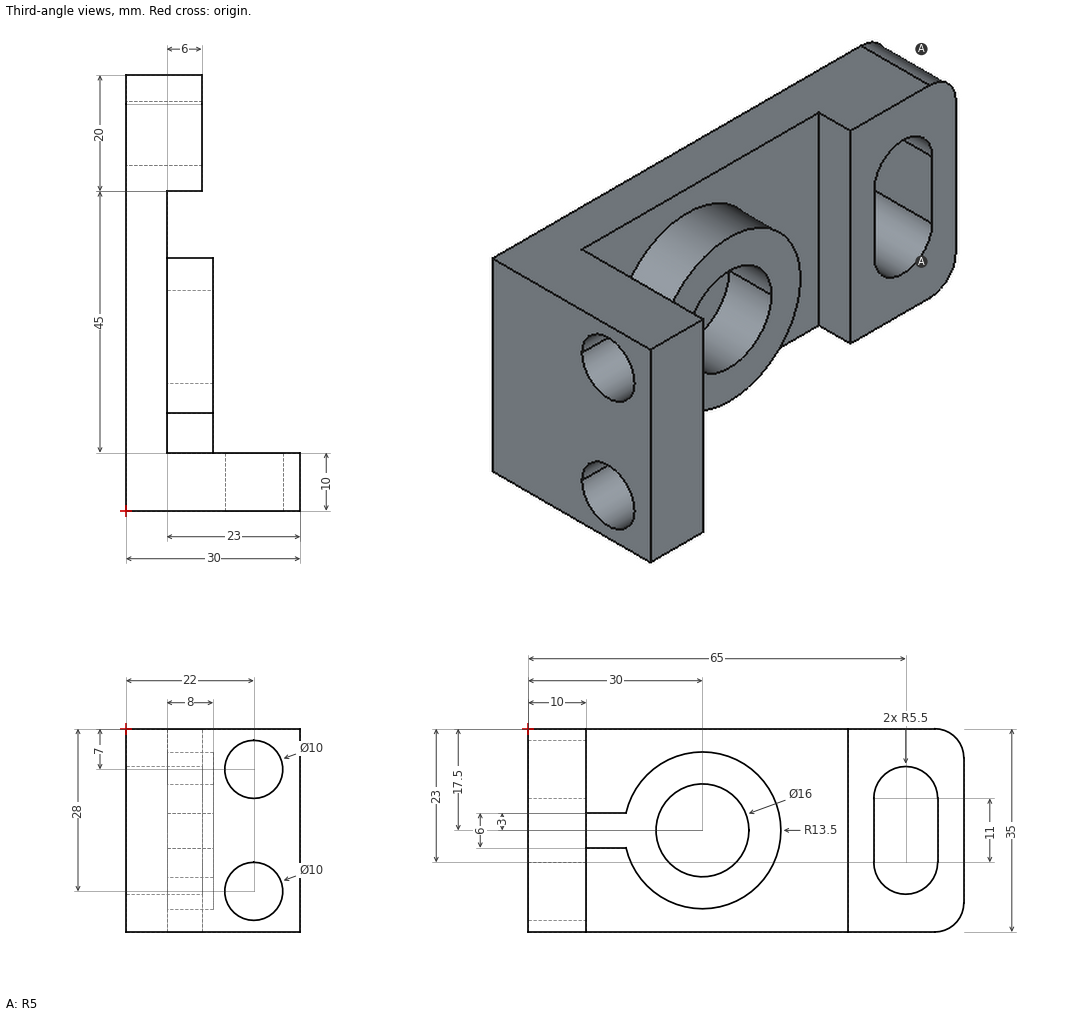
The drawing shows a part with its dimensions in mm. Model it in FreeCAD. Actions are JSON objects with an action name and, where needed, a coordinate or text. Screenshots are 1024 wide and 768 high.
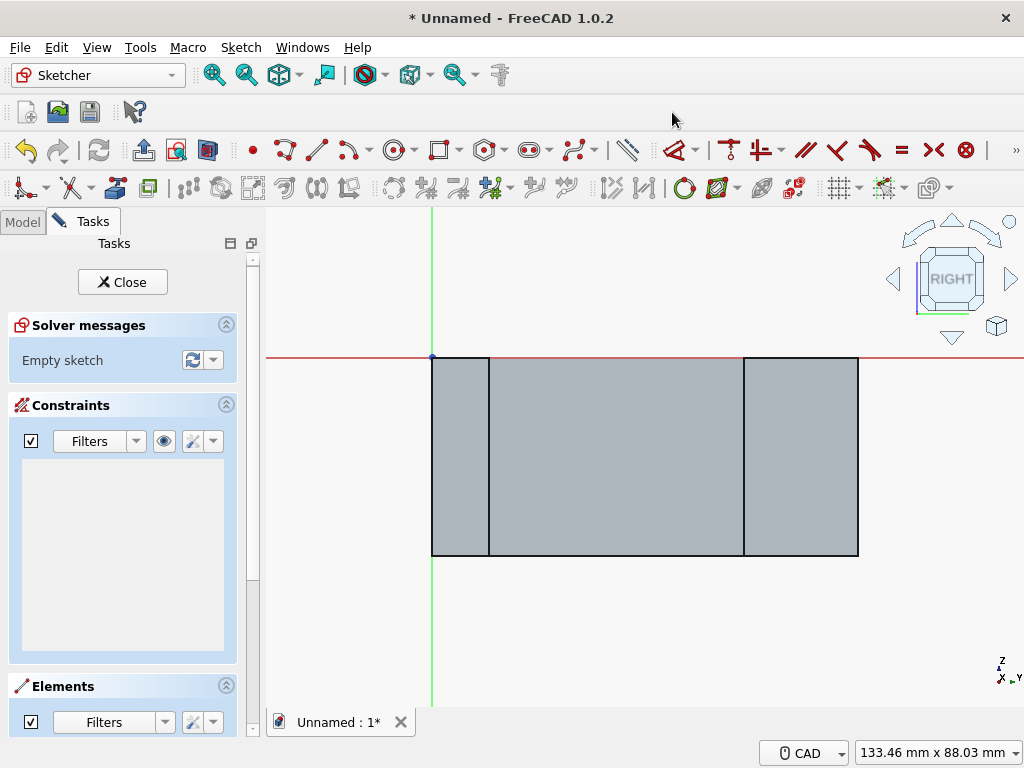
{"action": "scroll", "coordinate": [513, 375], "scroll_direction": "up", "scroll_amount": 2}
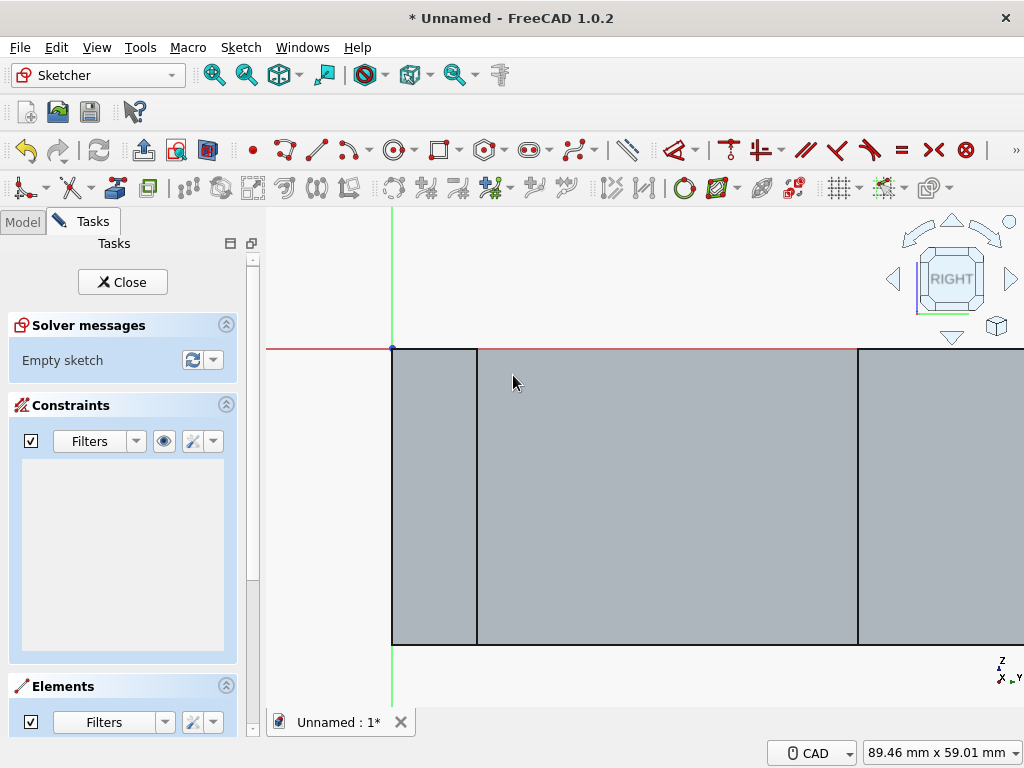
{"action": "left_click", "coordinate": [286, 150]}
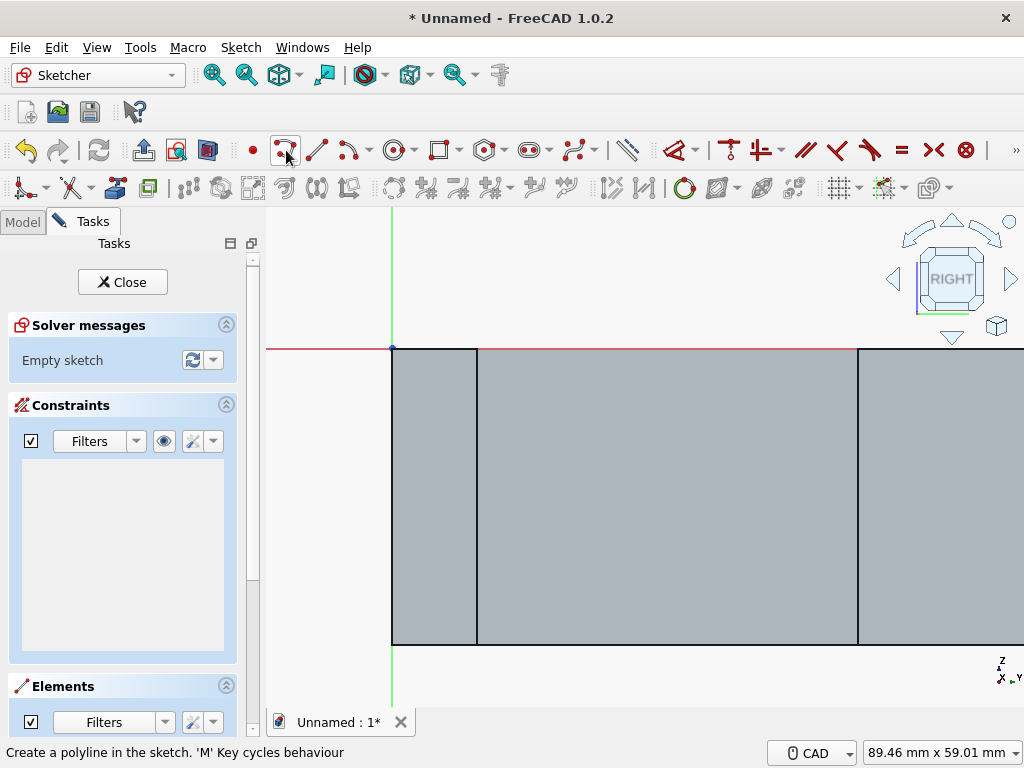
{"action": "left_click", "coordinate": [535, 472]}
{"action": "left_click", "coordinate": [477, 472]}
{"action": "left_click", "coordinate": [477, 523]}
{"action": "left_click", "coordinate": [535, 523]}
{"action": "right_click", "coordinate": [535, 523]}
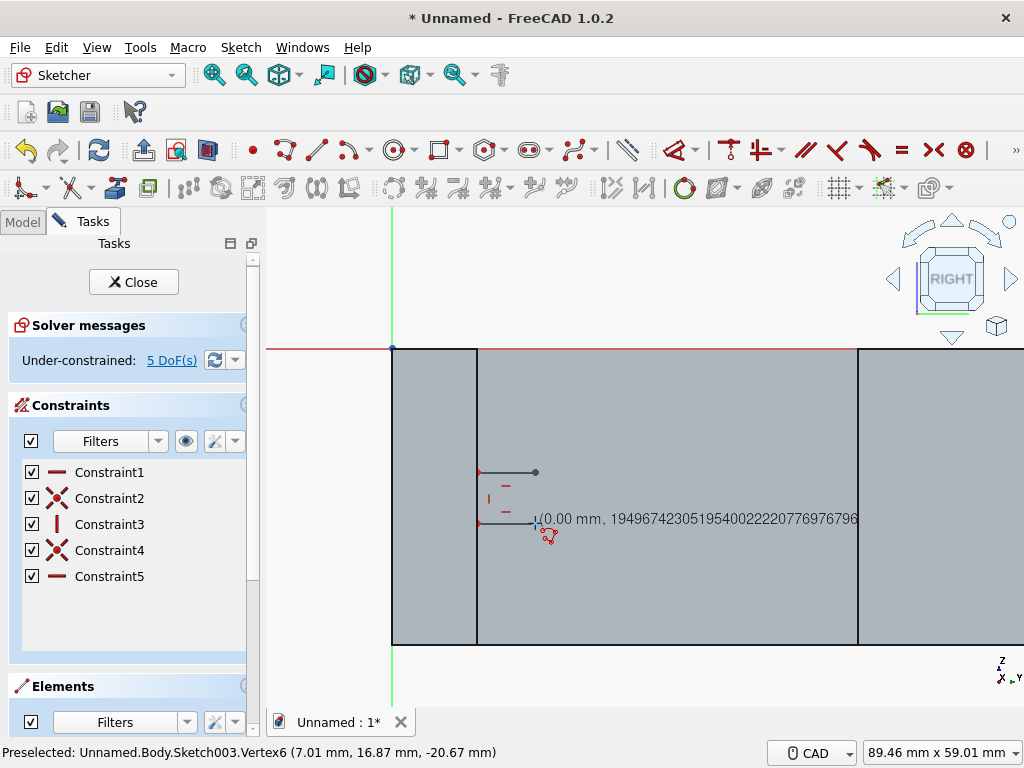
{"action": "key", "text": "g 3 a"}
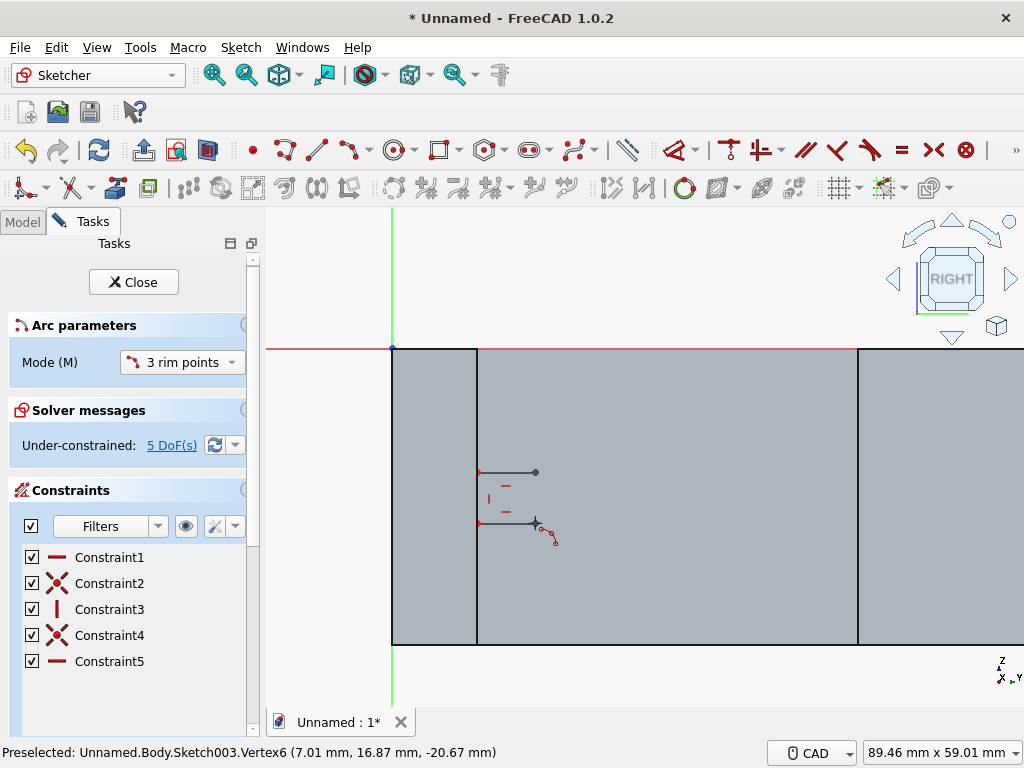
{"action": "left_click", "coordinate": [535, 524]}
{"action": "left_click", "coordinate": [535, 473]}
{"action": "left_click", "coordinate": [761, 497]}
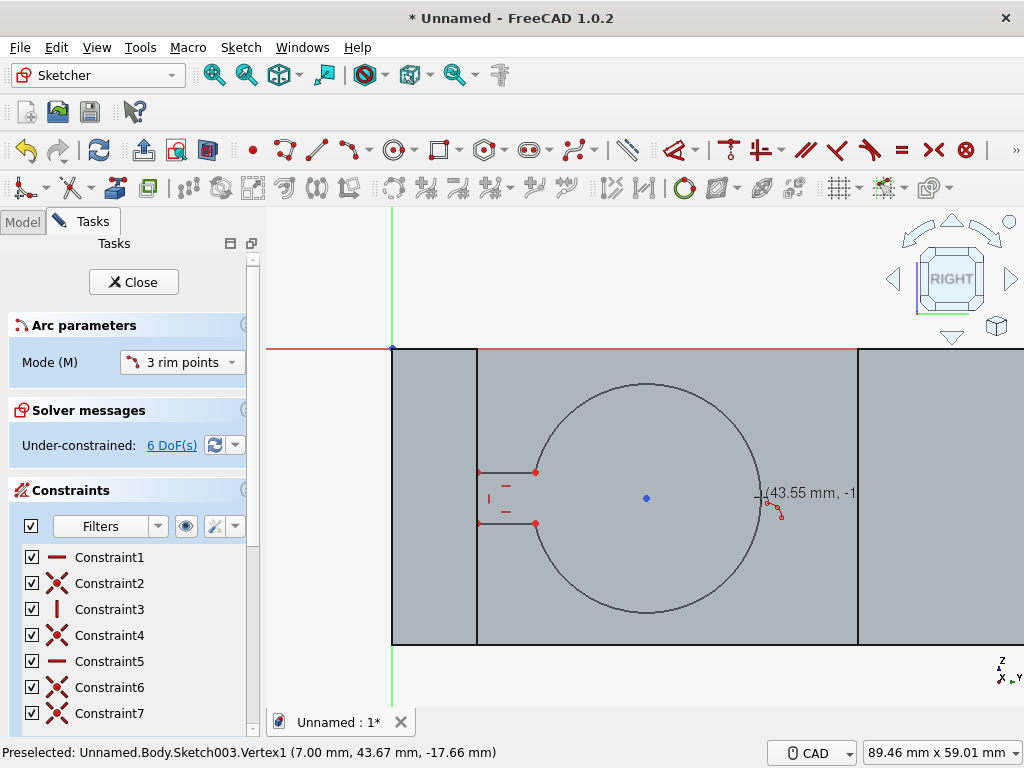
{"action": "left_click", "coordinate": [394, 150]}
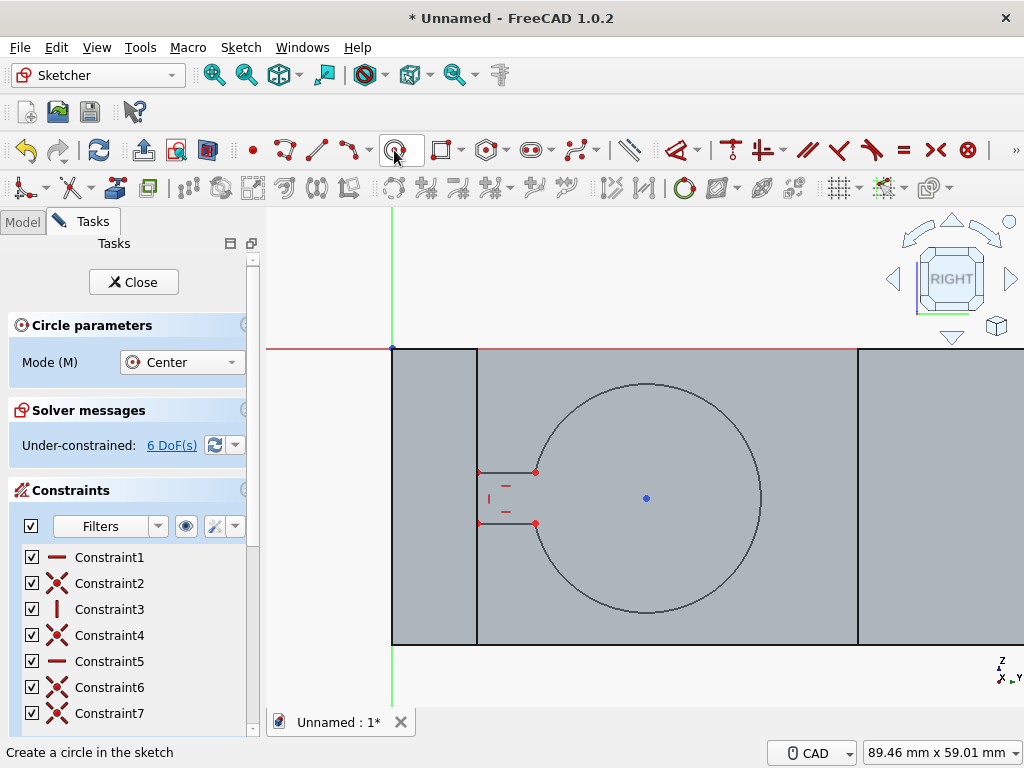
{"action": "left_click", "coordinate": [646, 497]}
{"action": "left_click", "coordinate": [694, 449]}
{"action": "key", "text": "Escape"}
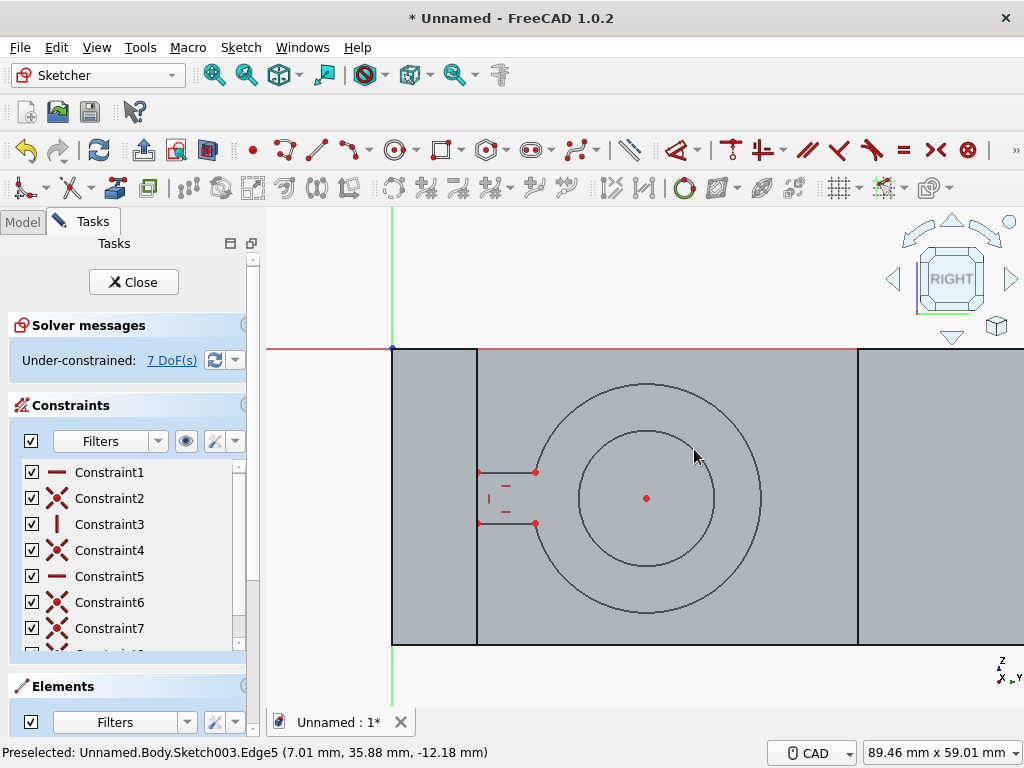
{"action": "key", "text": "d"}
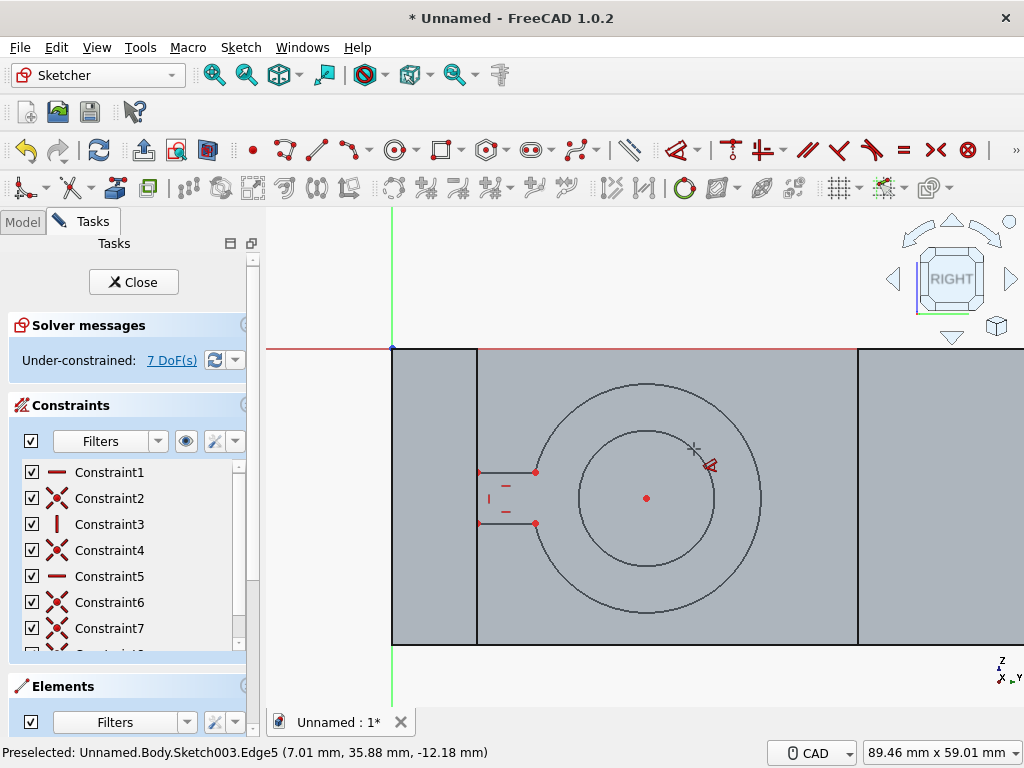
{"action": "left_click", "coordinate": [692, 604]}
{"action": "left_click", "coordinate": [705, 633]}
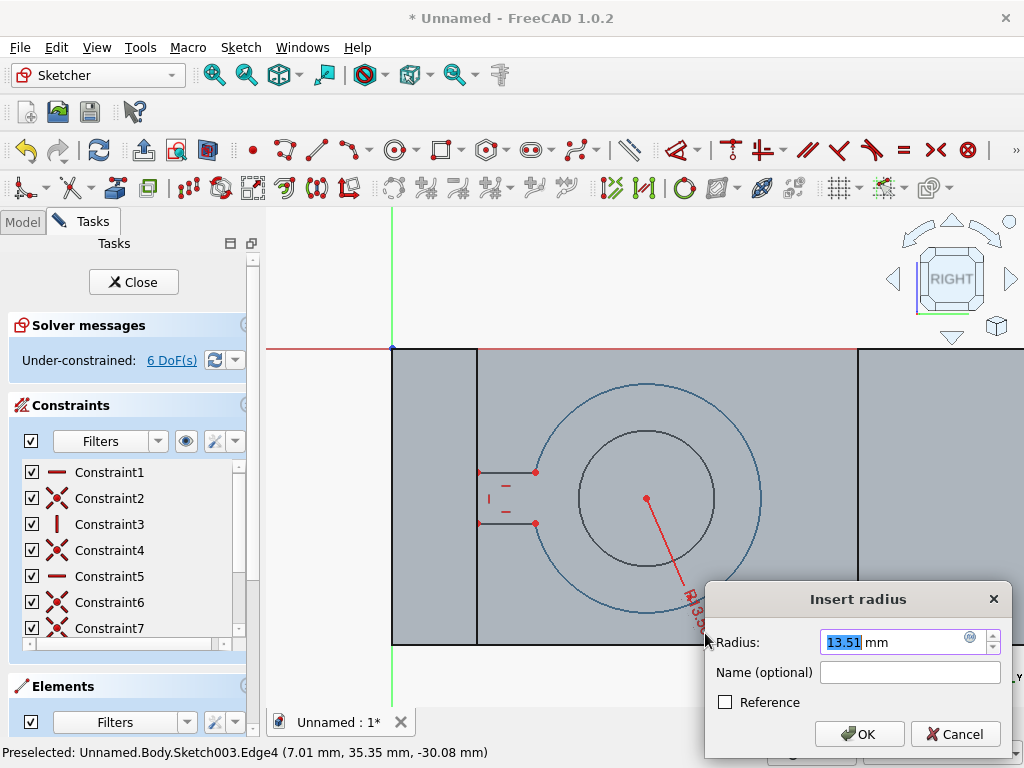
{"action": "type", "text": "13.5"}
{"action": "key", "text": "Return"}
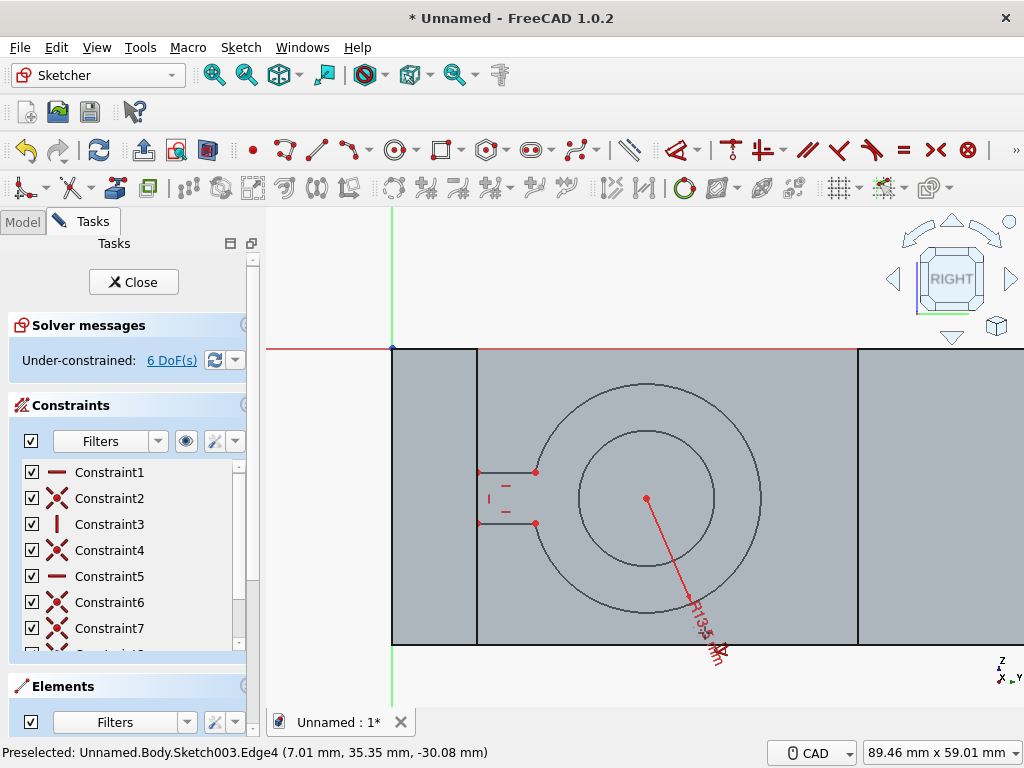
{"action": "left_click", "coordinate": [694, 450]}
{"action": "left_click", "coordinate": [716, 427]}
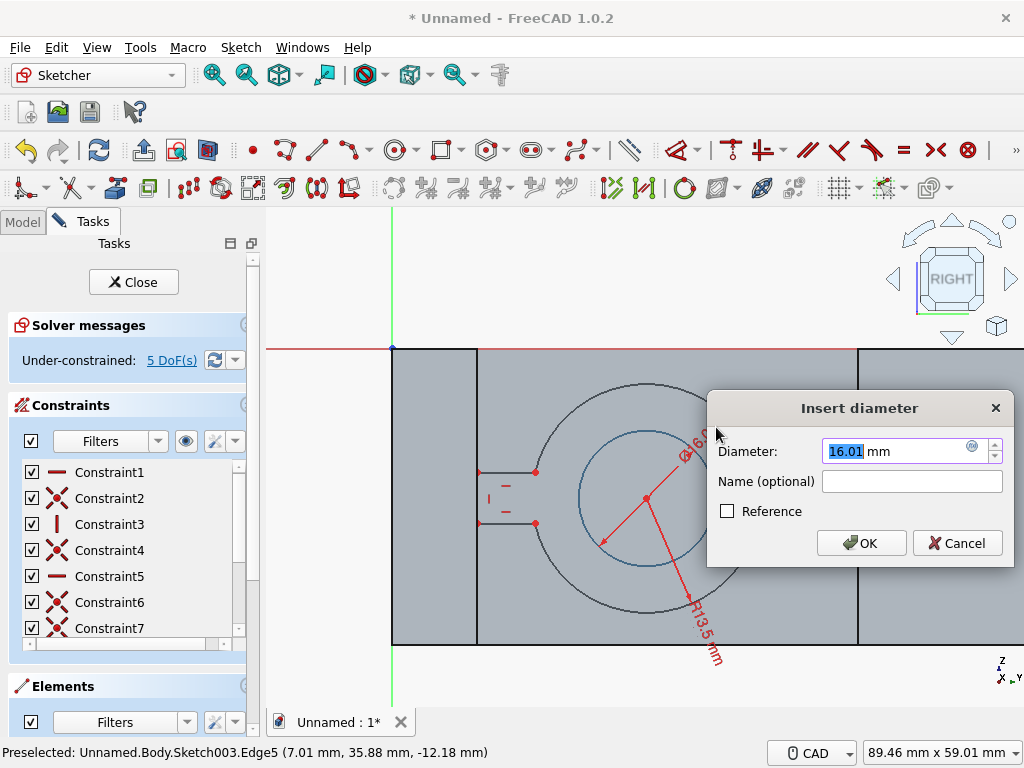
{"action": "type", "text": "16"}
{"action": "key", "text": "Return"}